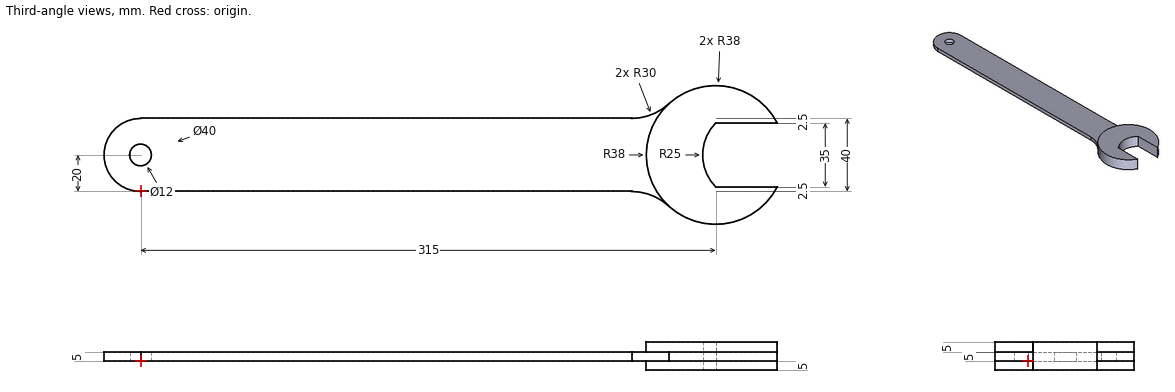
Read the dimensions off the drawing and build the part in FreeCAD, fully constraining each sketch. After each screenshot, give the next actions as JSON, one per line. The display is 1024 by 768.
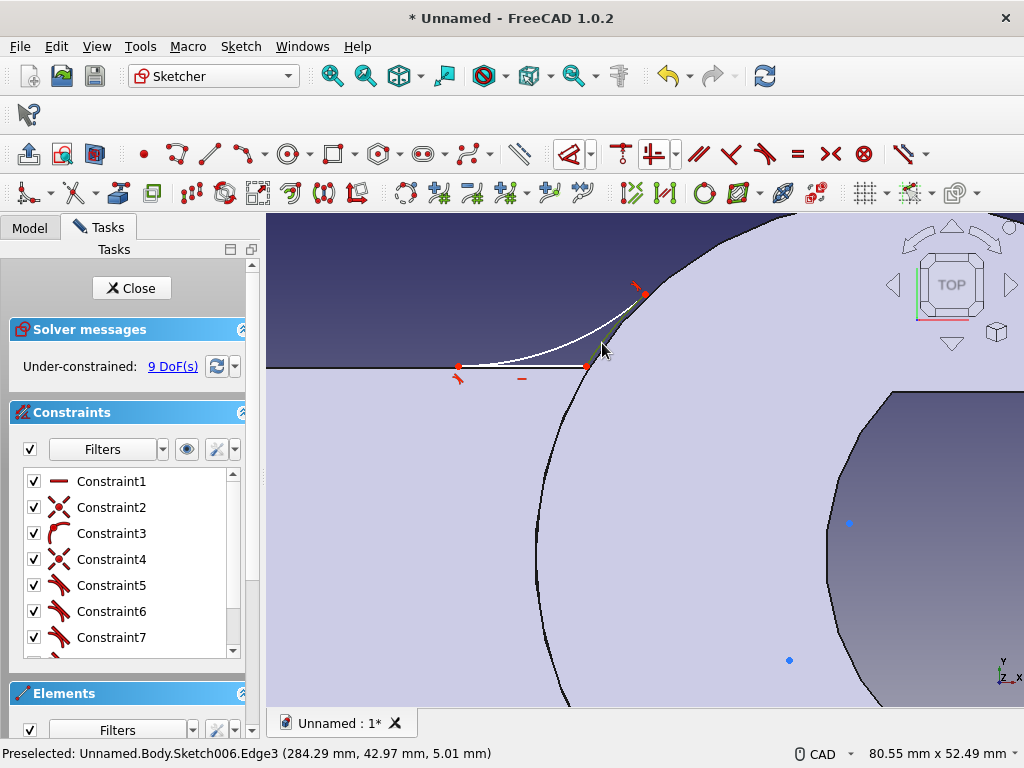
{"action": "scroll", "coordinate": [603, 343], "scroll_direction": "down", "scroll_amount": 3}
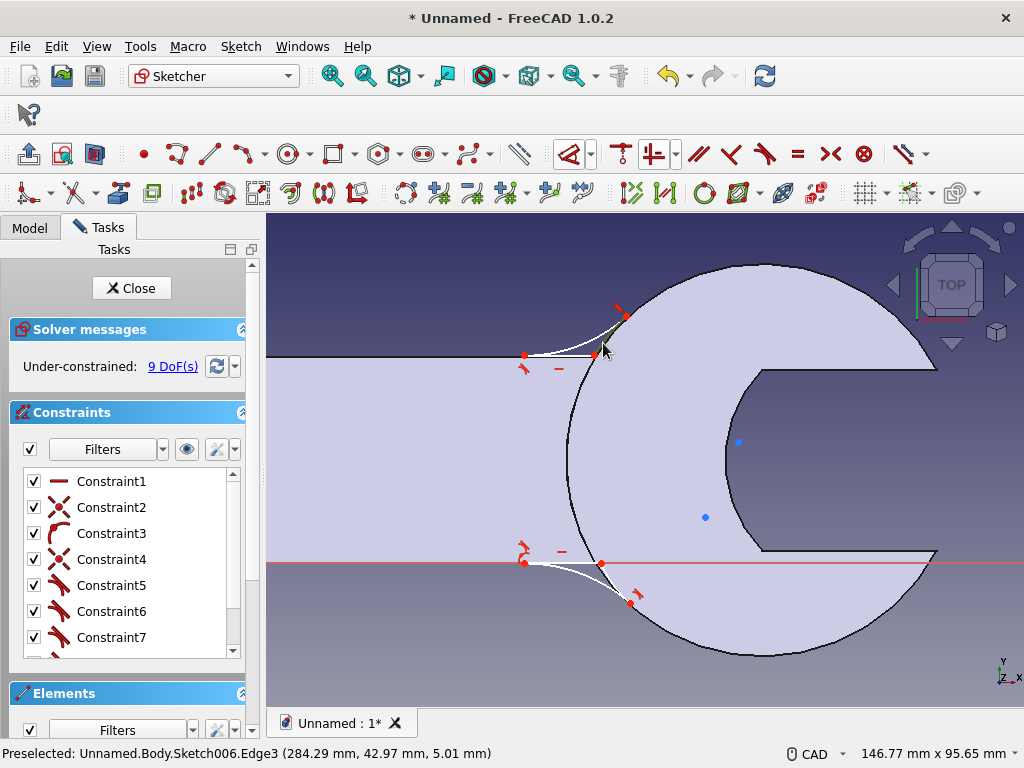
{"action": "scroll", "coordinate": [608, 577], "scroll_direction": "up", "scroll_amount": 3}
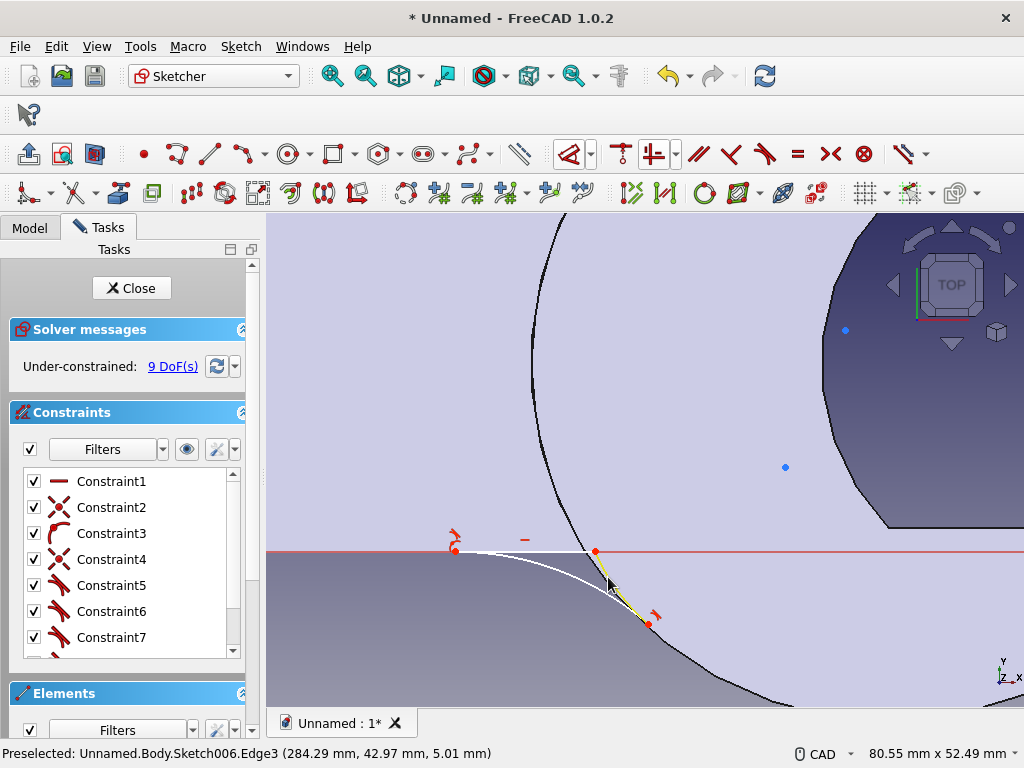
{"action": "left_click", "coordinate": [608, 576]}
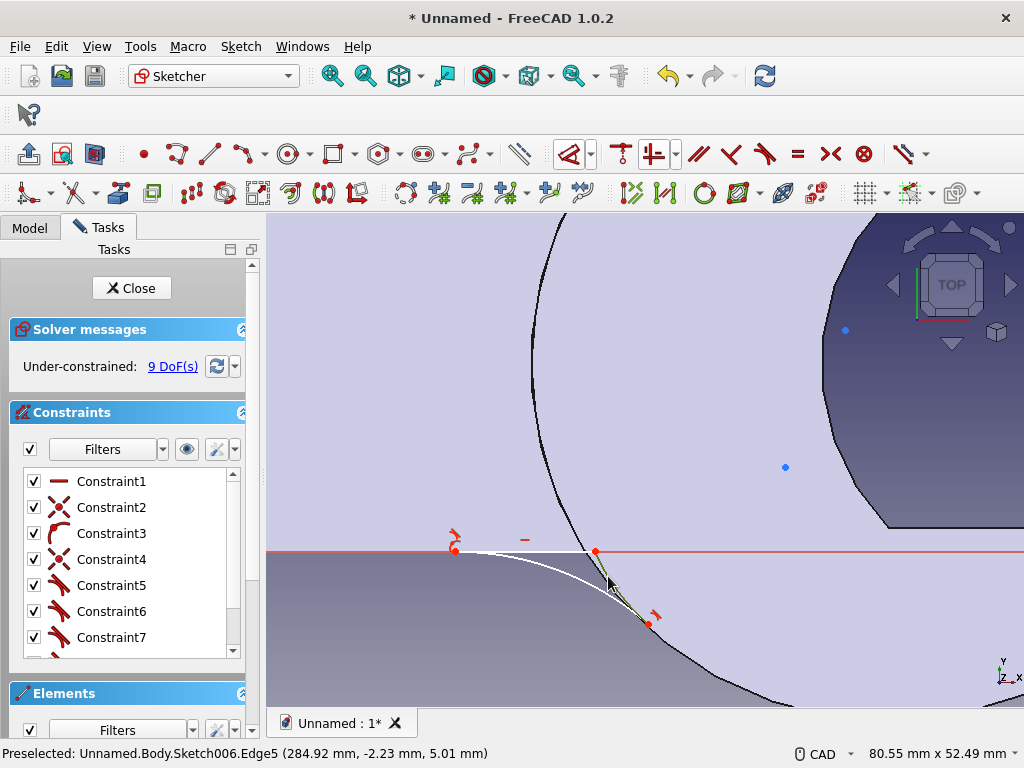
{"action": "left_click", "coordinate": [621, 154]}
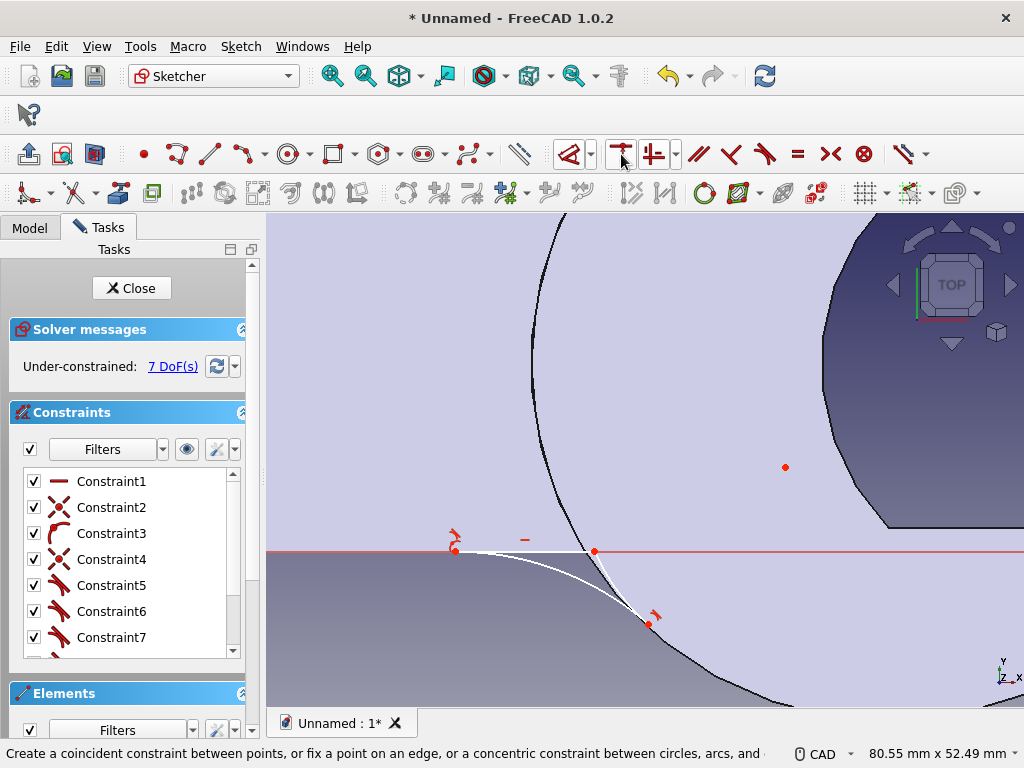
{"action": "scroll", "coordinate": [608, 577], "scroll_direction": "down", "scroll_amount": 3}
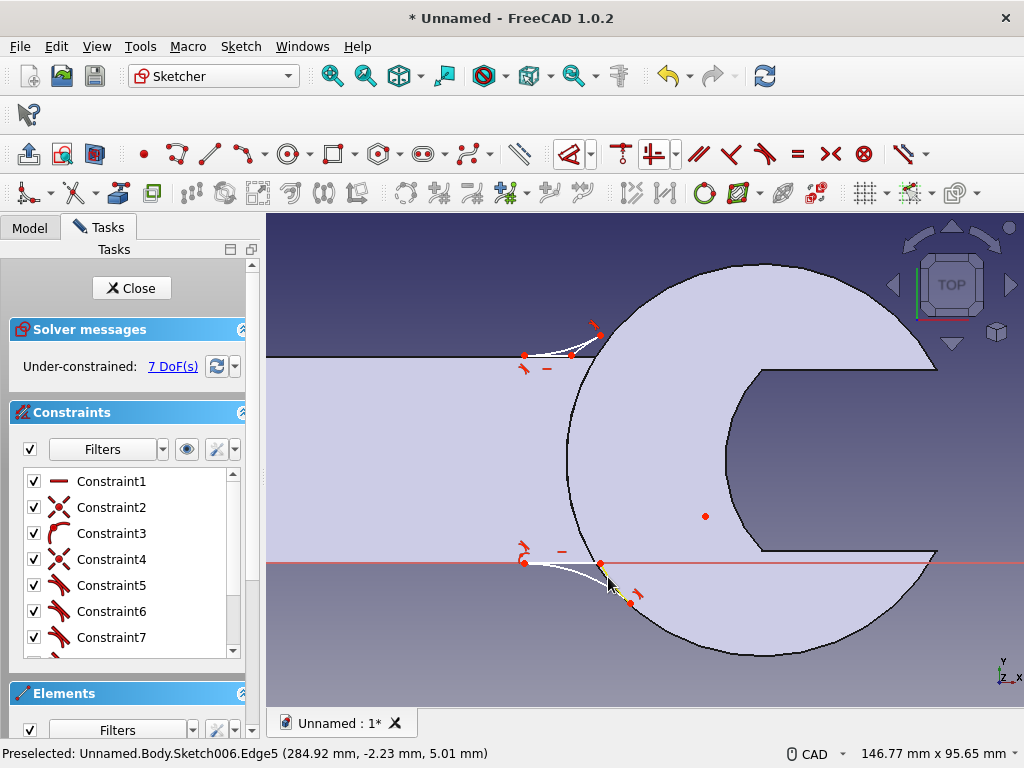
{"action": "scroll", "coordinate": [577, 351], "scroll_direction": "up", "scroll_amount": 6}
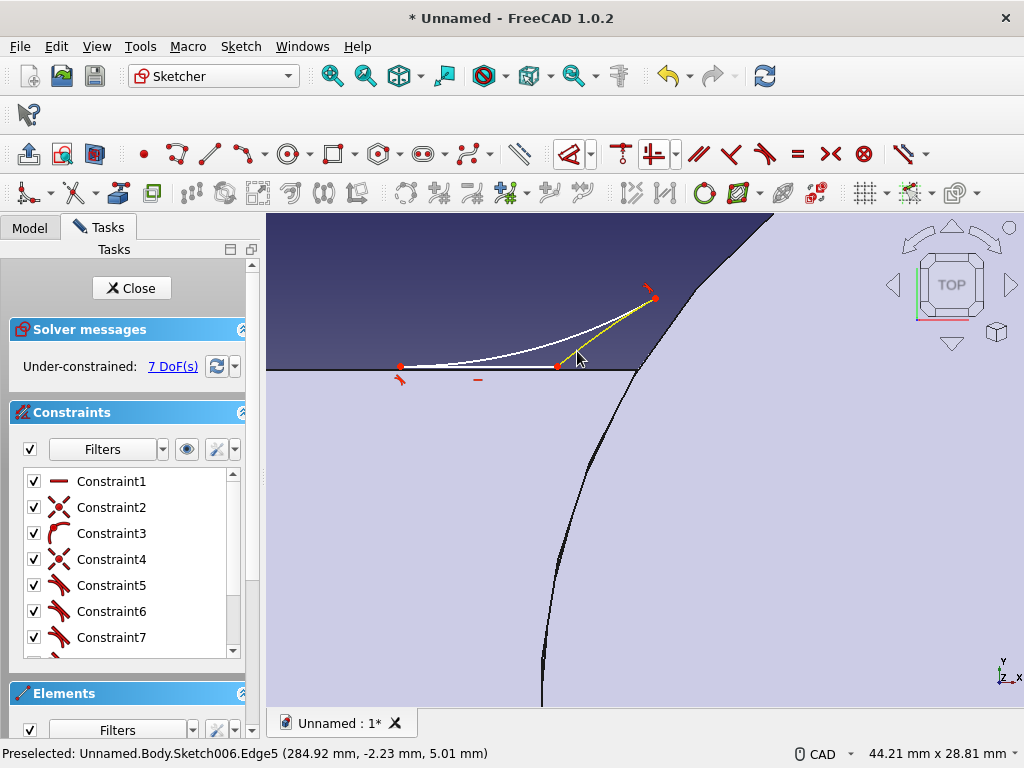
{"action": "left_click", "coordinate": [576, 352]}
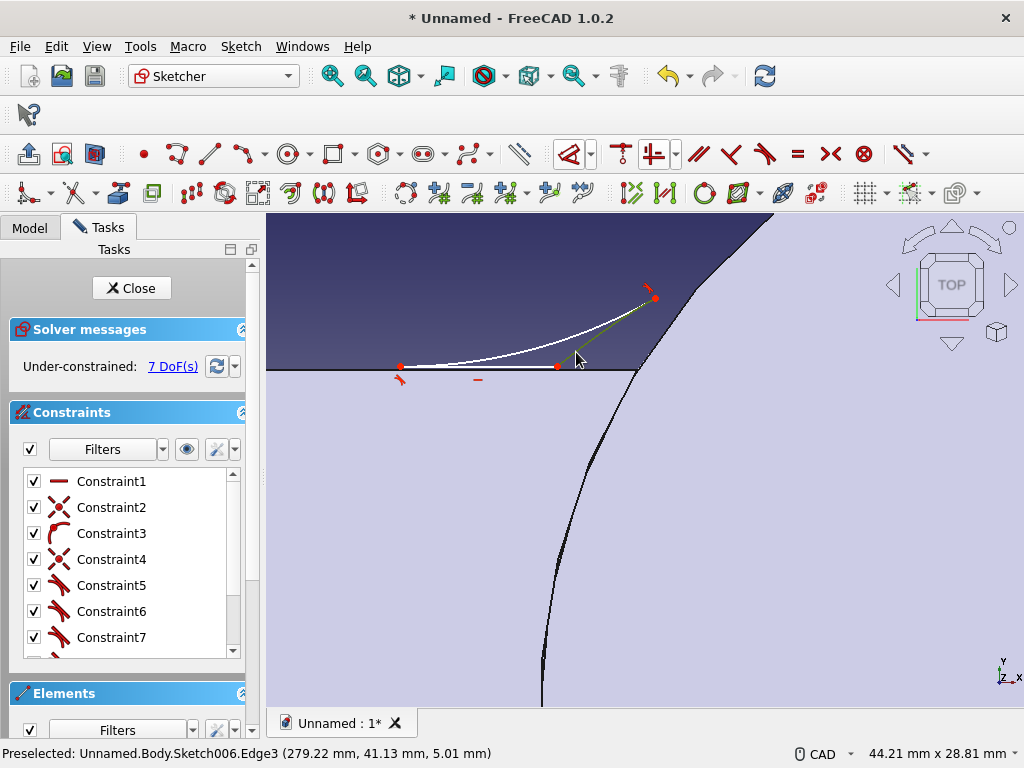
{"action": "scroll", "coordinate": [577, 351], "scroll_direction": "down", "scroll_amount": 6}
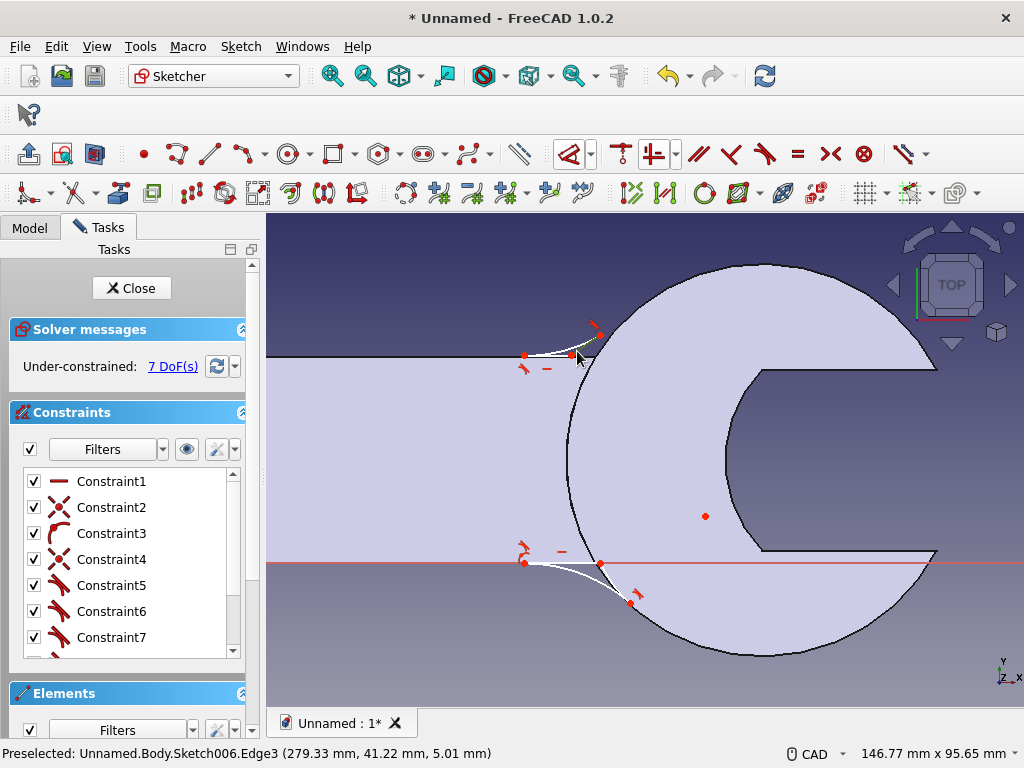
{"action": "scroll", "coordinate": [608, 577], "scroll_direction": "up", "scroll_amount": 3}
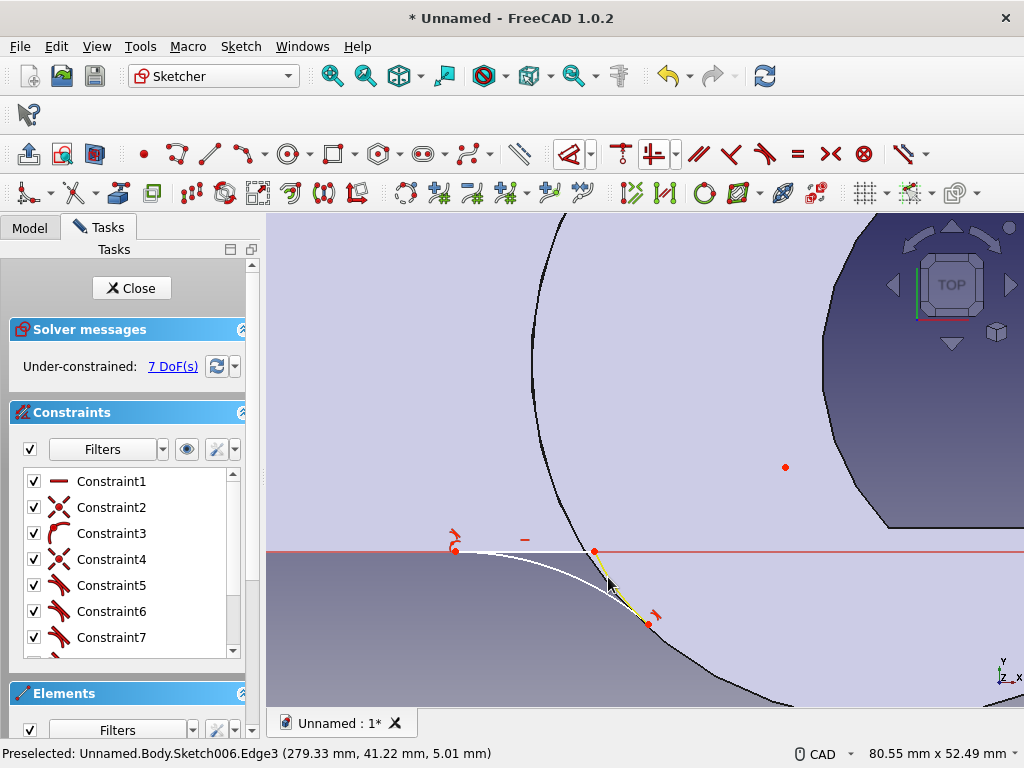
{"action": "left_click", "coordinate": [607, 576]}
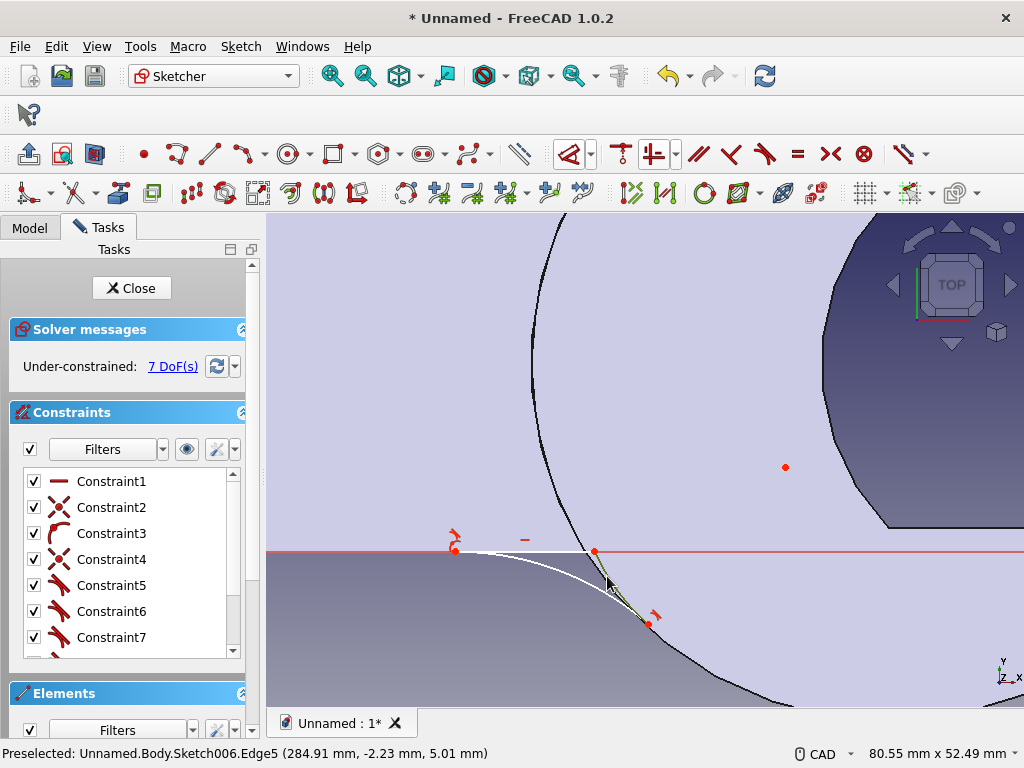
{"action": "left_click", "coordinate": [798, 154]}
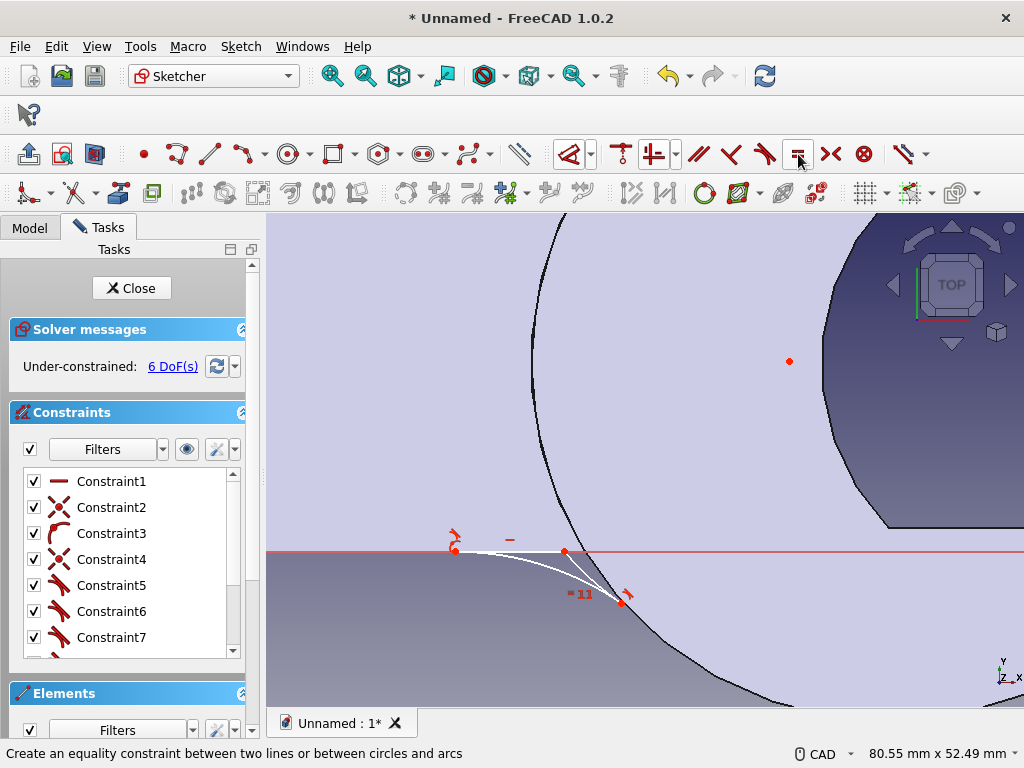
{"action": "scroll", "coordinate": [608, 577], "scroll_direction": "down", "scroll_amount": 3}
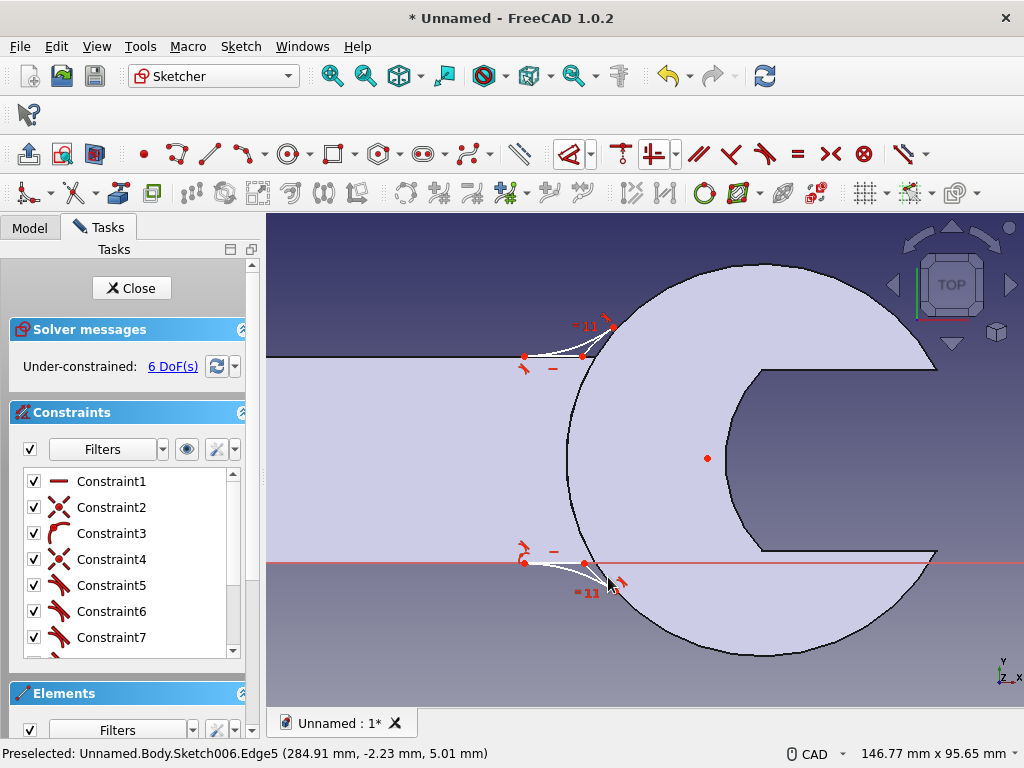
{"action": "scroll", "coordinate": [589, 342], "scroll_direction": "up", "scroll_amount": 5}